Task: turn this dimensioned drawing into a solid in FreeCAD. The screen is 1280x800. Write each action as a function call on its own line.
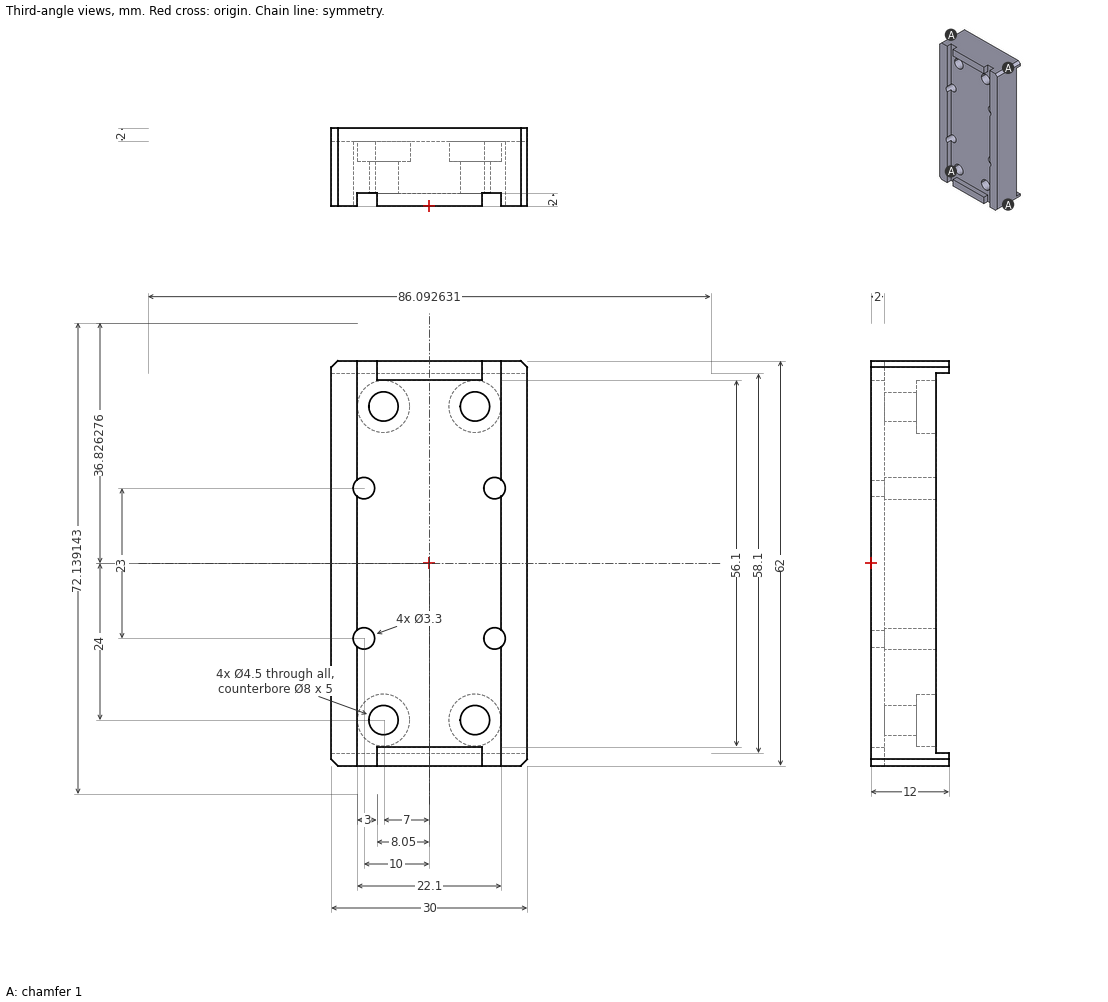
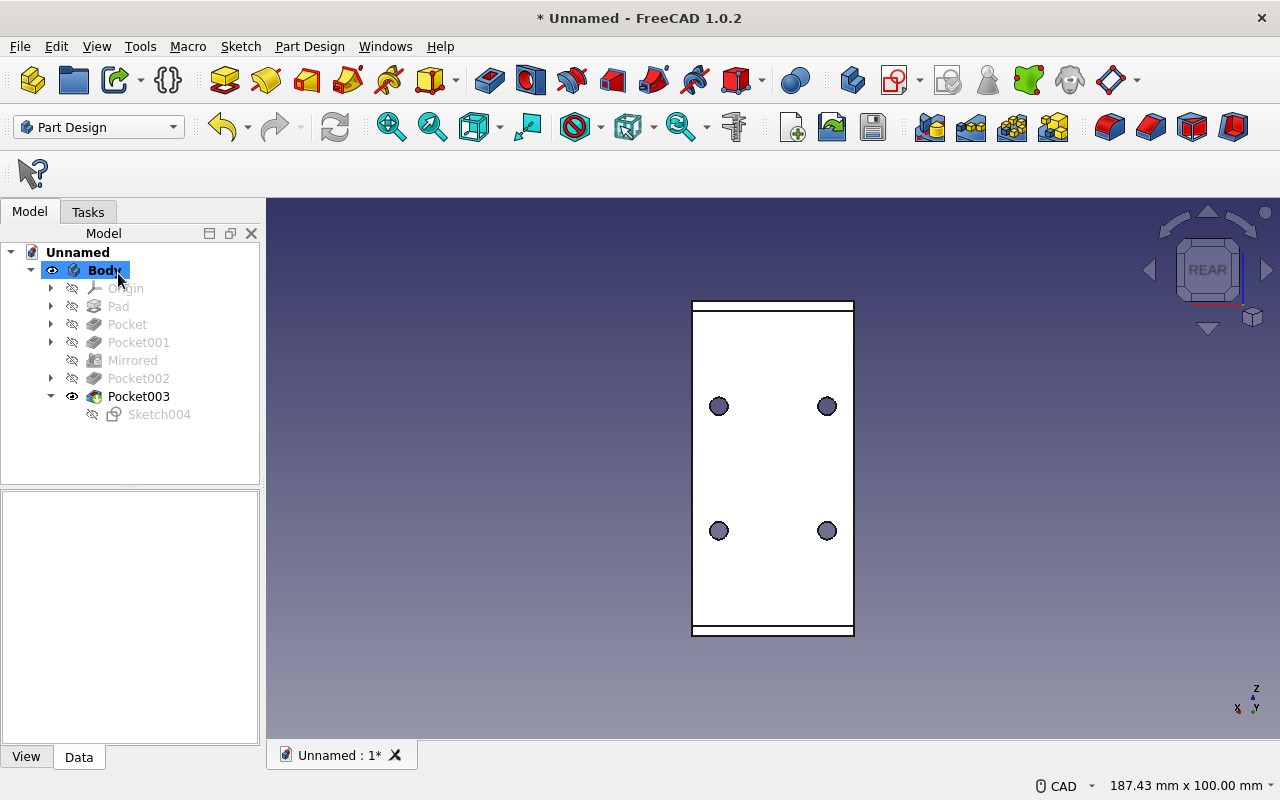
scroll(703, 630, up, 5)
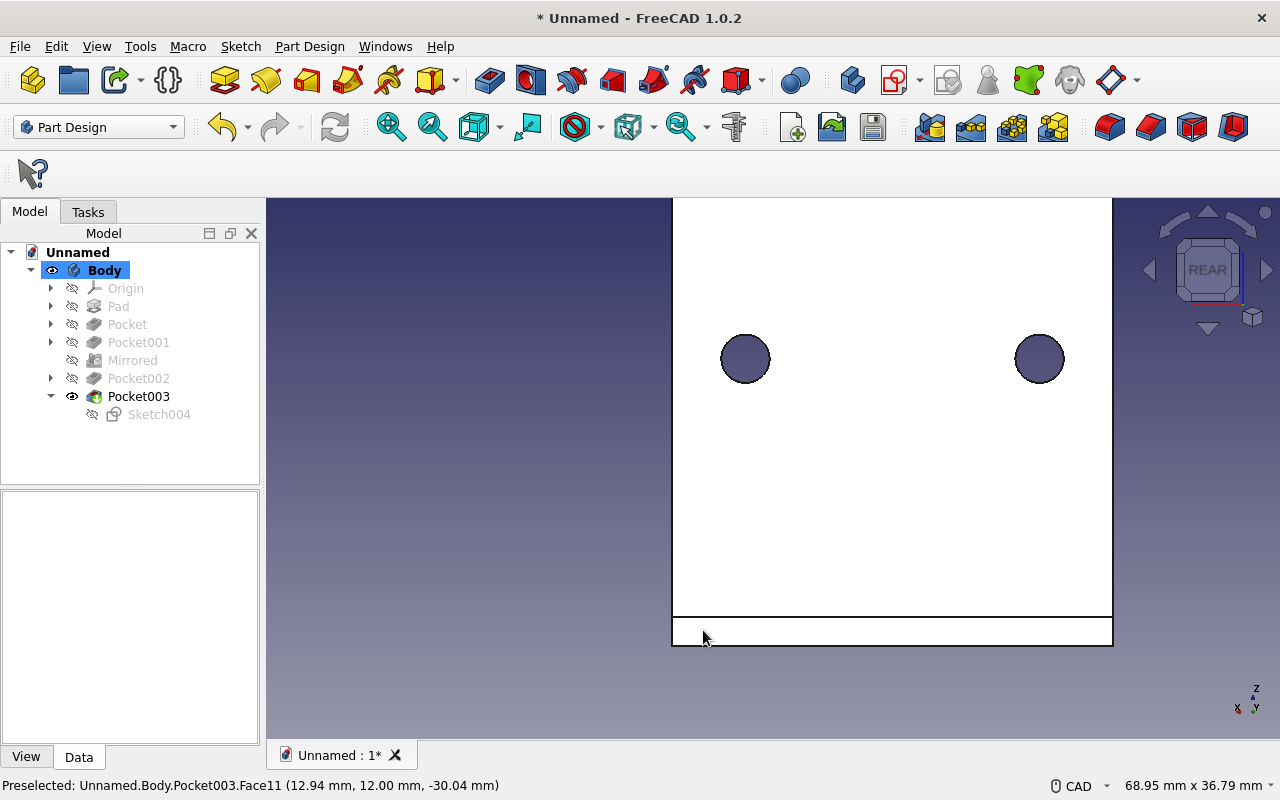
click(703, 630)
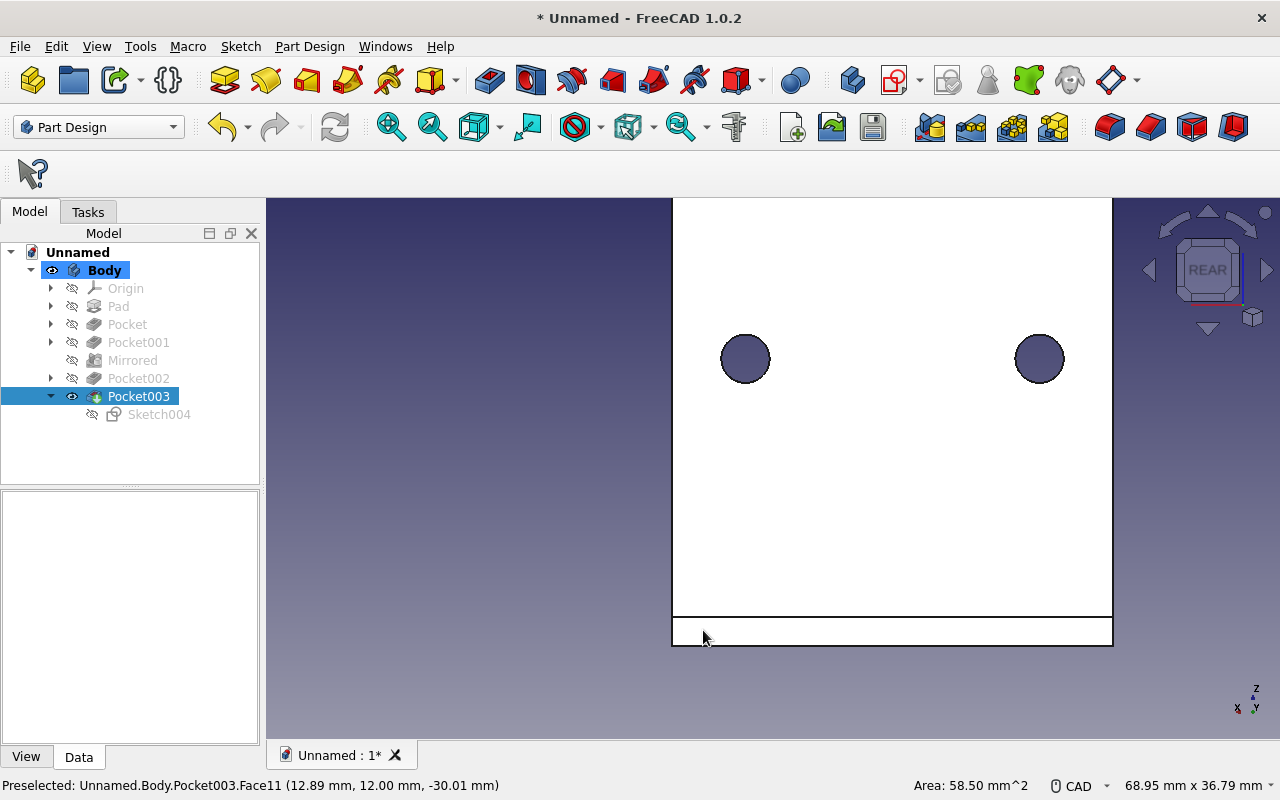
click(894, 80)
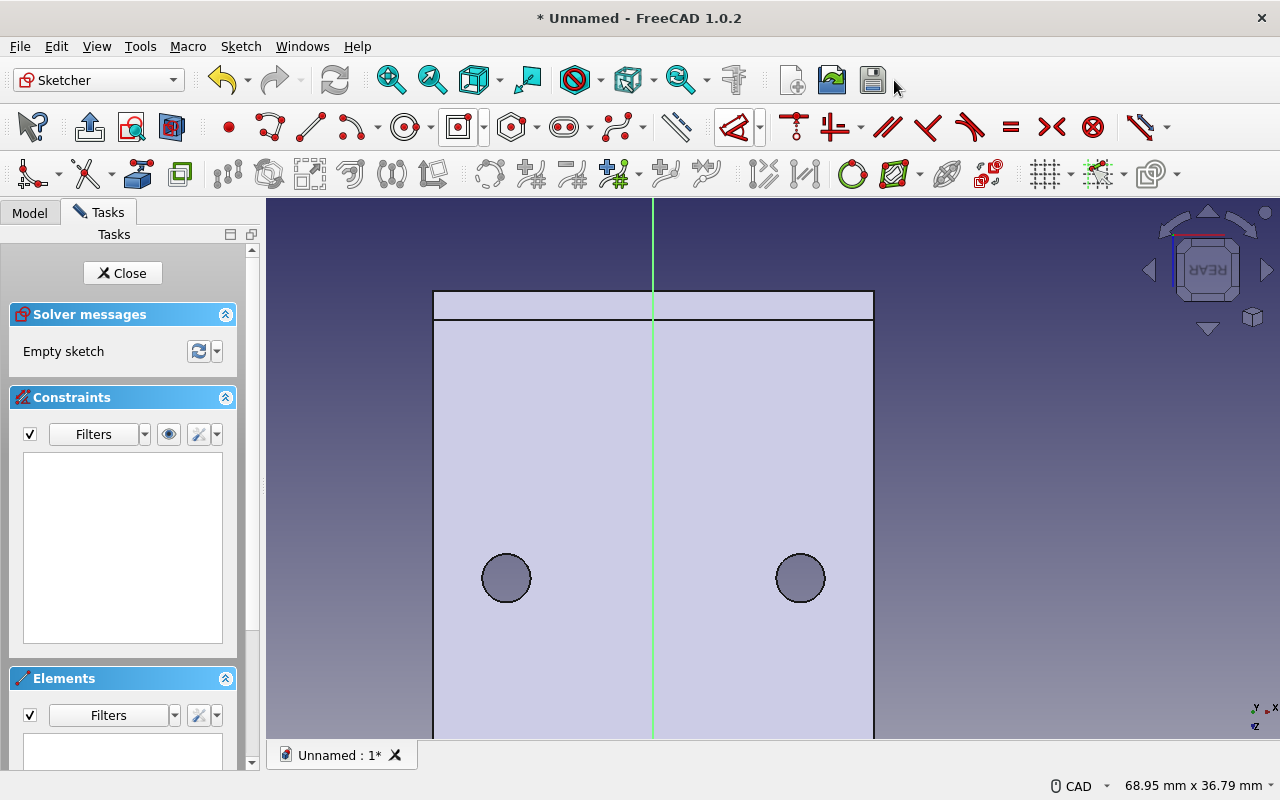
scroll(746, 241, down, 4)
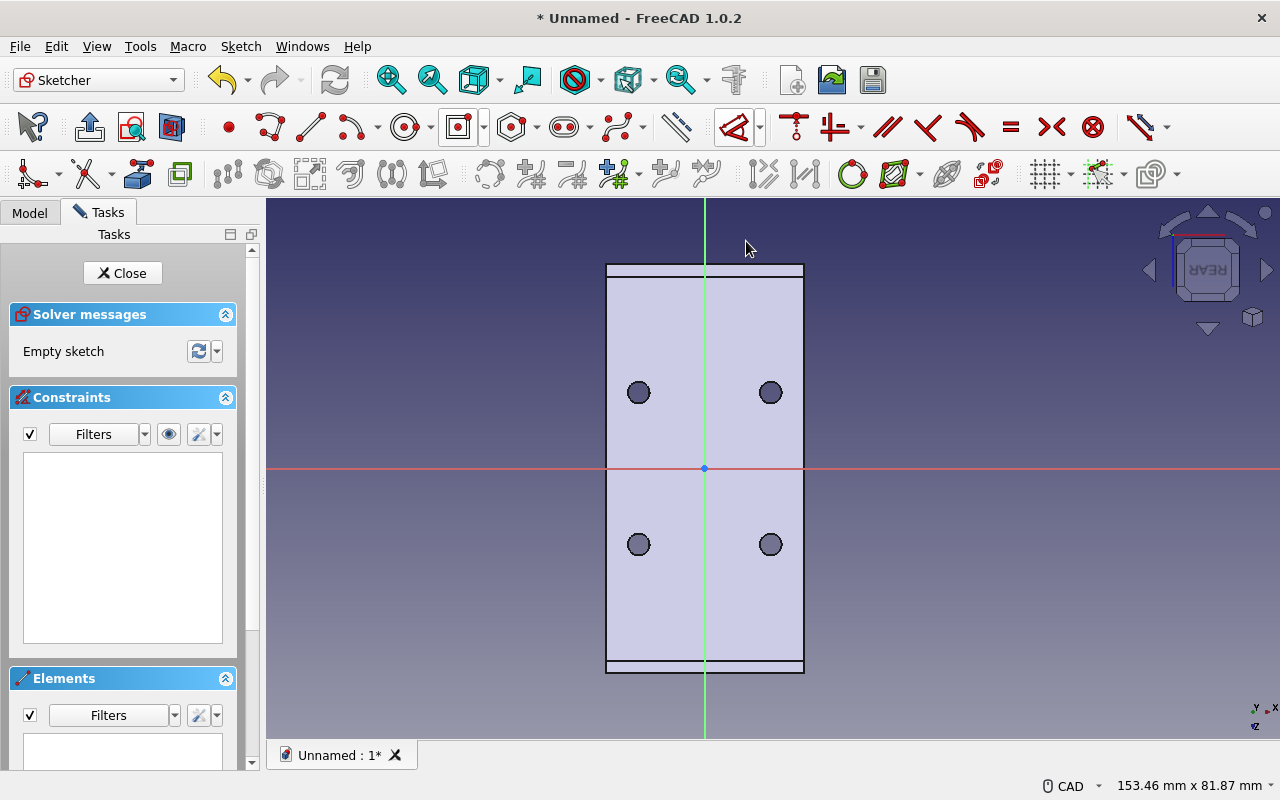
click(404, 128)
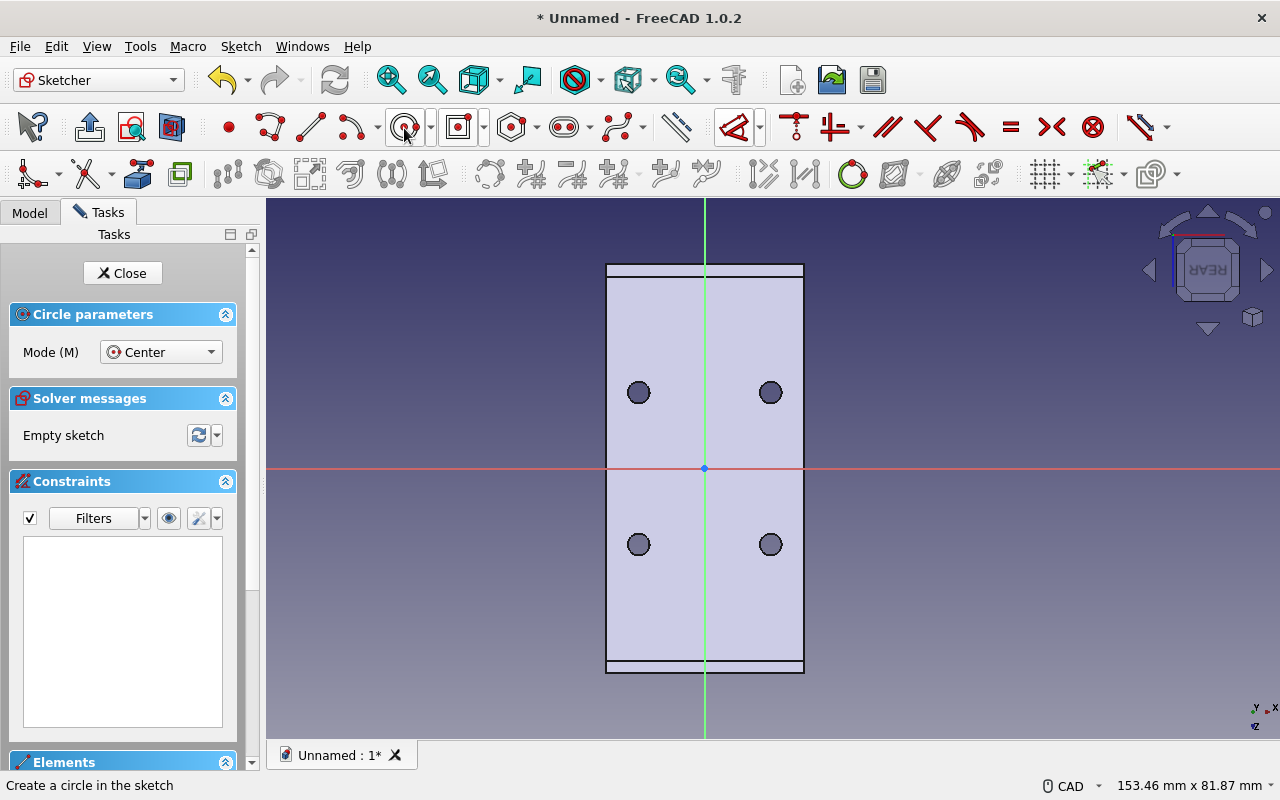
scroll(658, 310, up, 3)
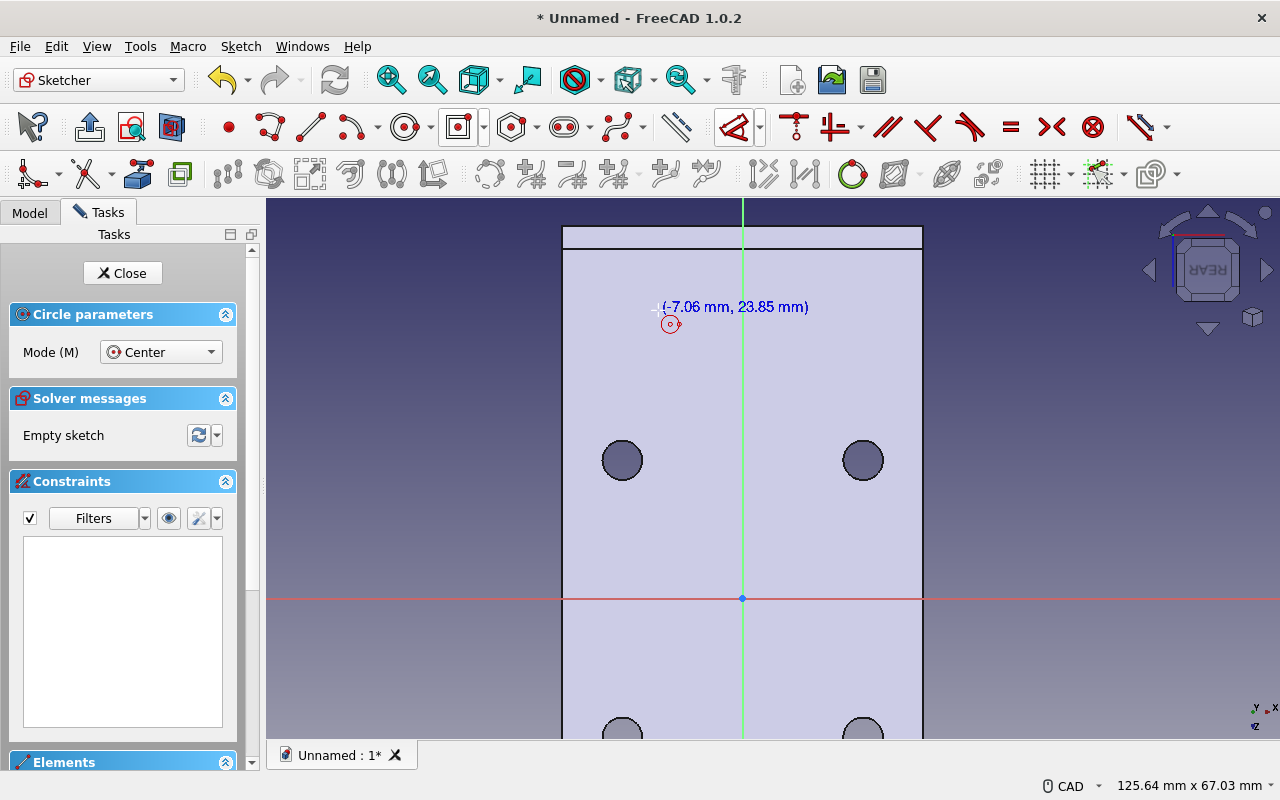
click(658, 310)
click(678, 291)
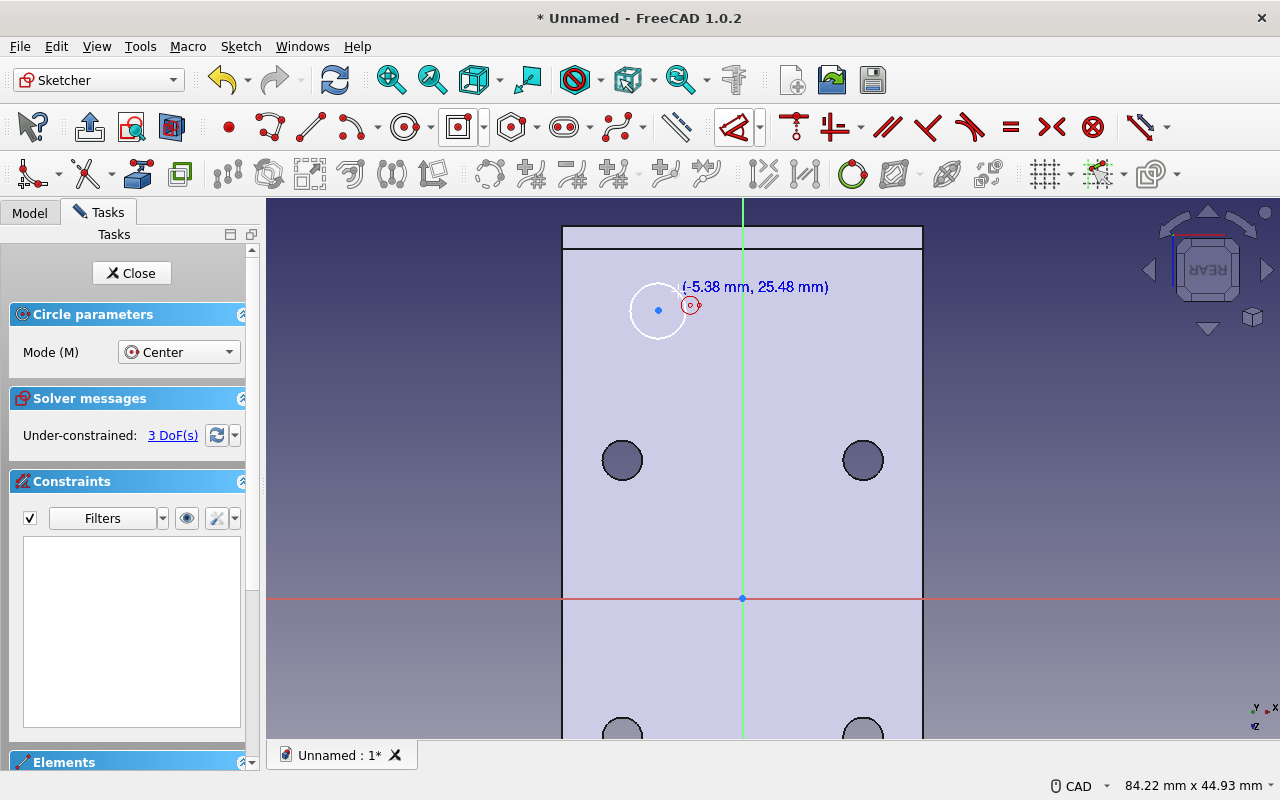
click(827, 310)
click(846, 291)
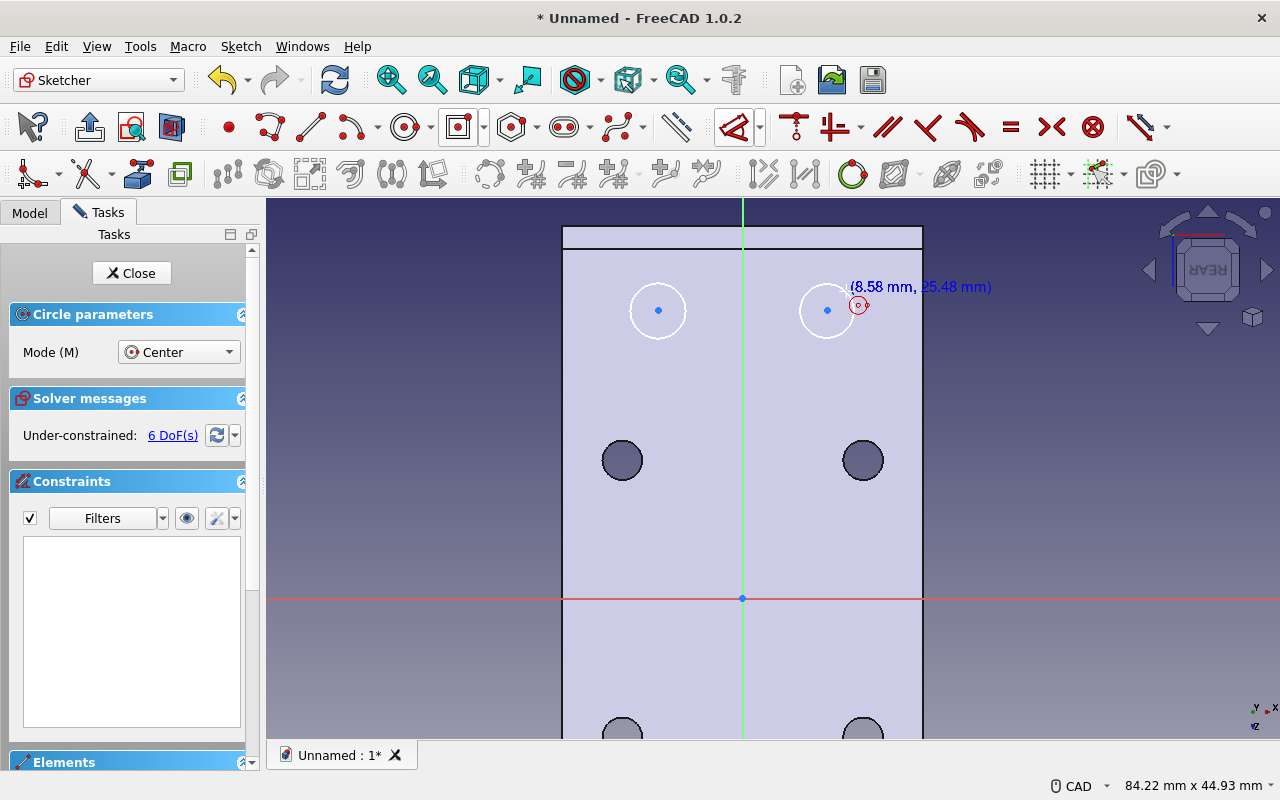
scroll(658, 310, down, 3)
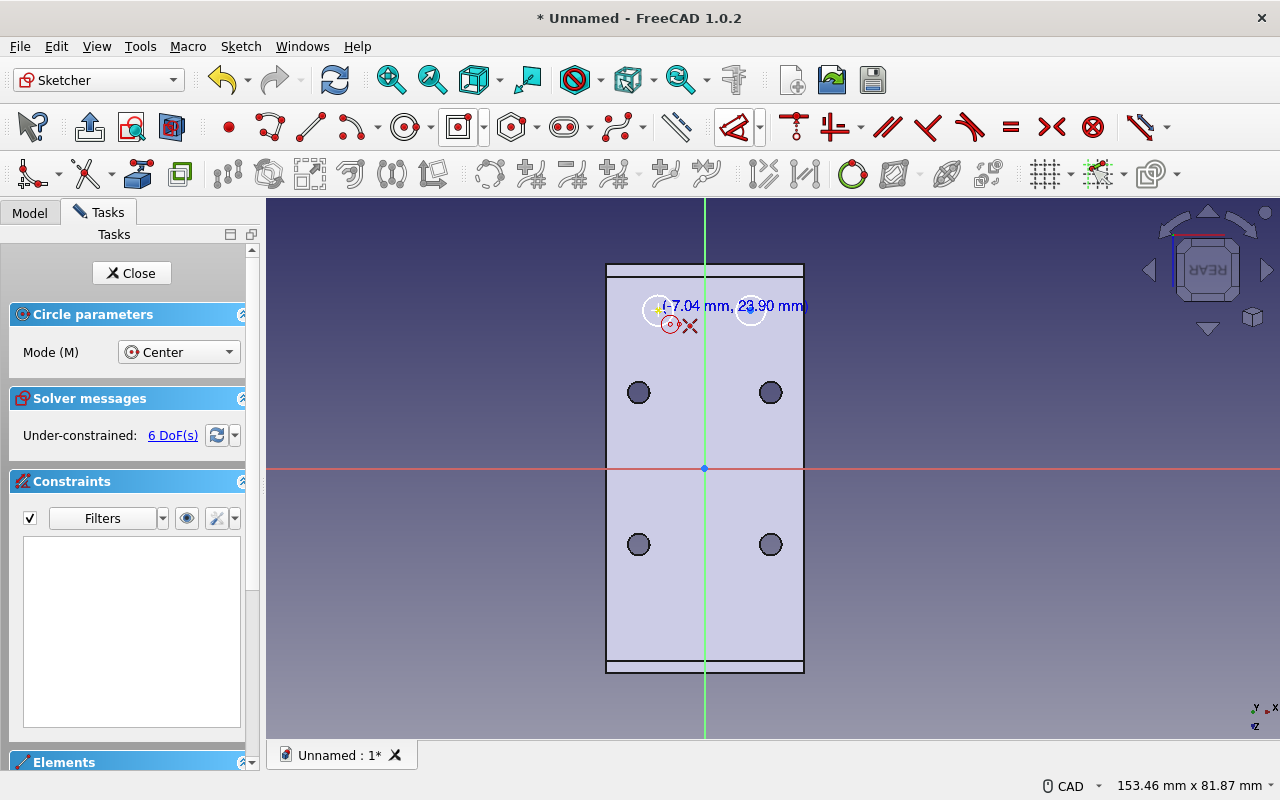
scroll(658, 627, up, 3)